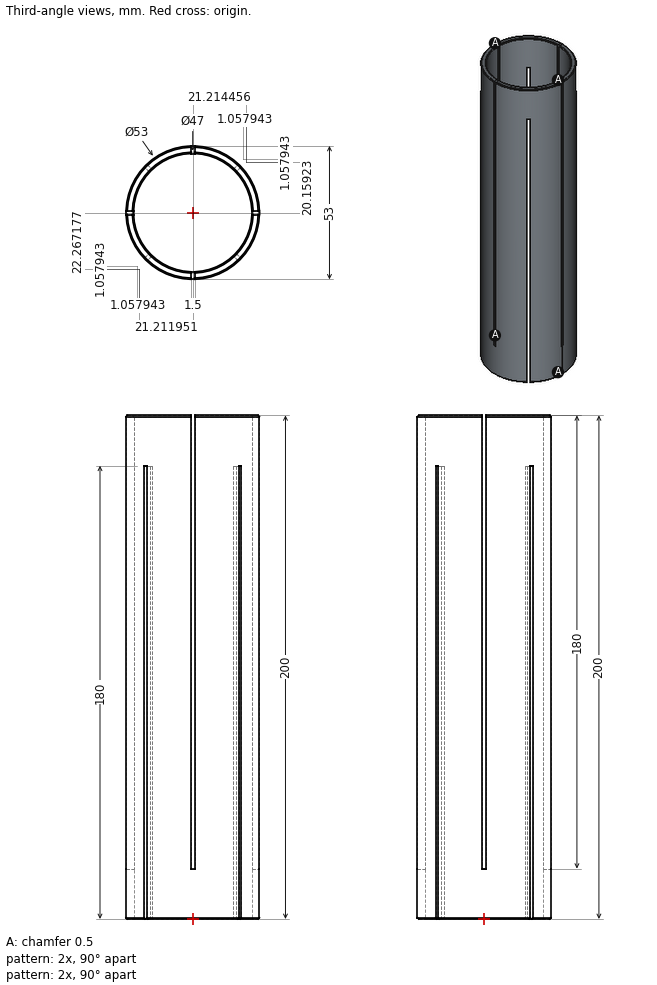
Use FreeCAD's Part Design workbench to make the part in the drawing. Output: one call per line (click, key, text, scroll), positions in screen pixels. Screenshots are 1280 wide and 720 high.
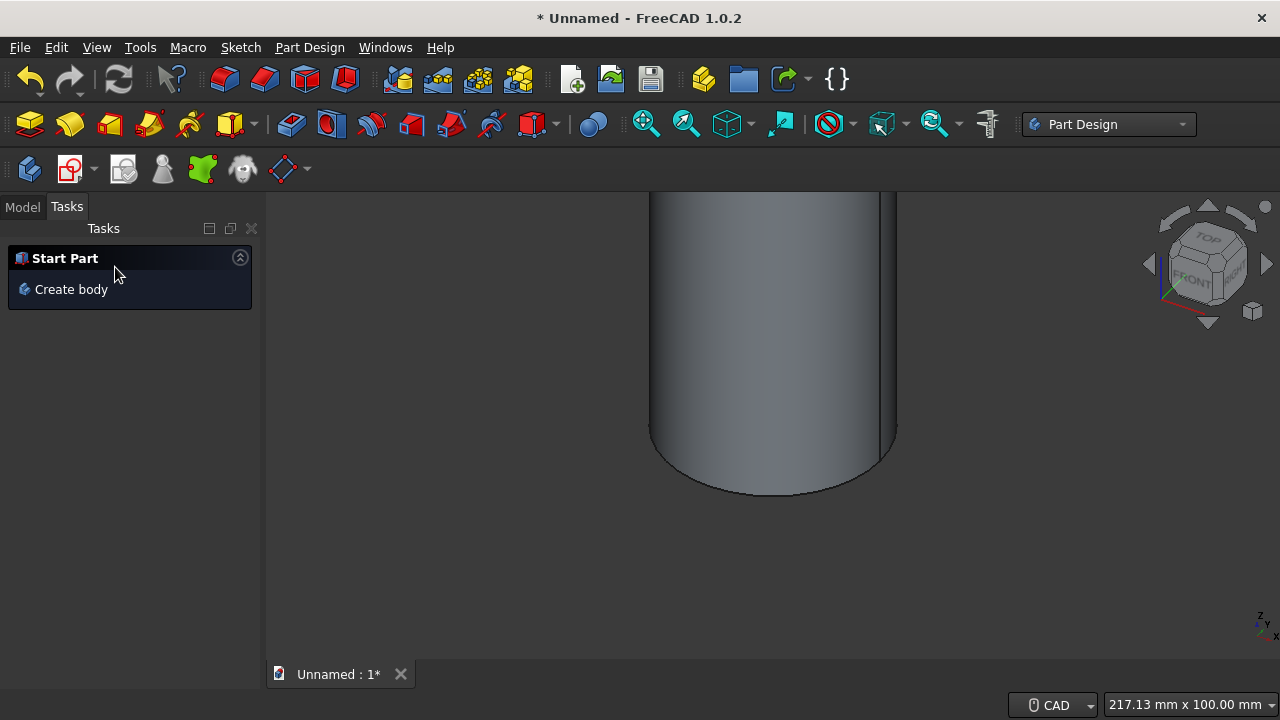
key(v)
key(f)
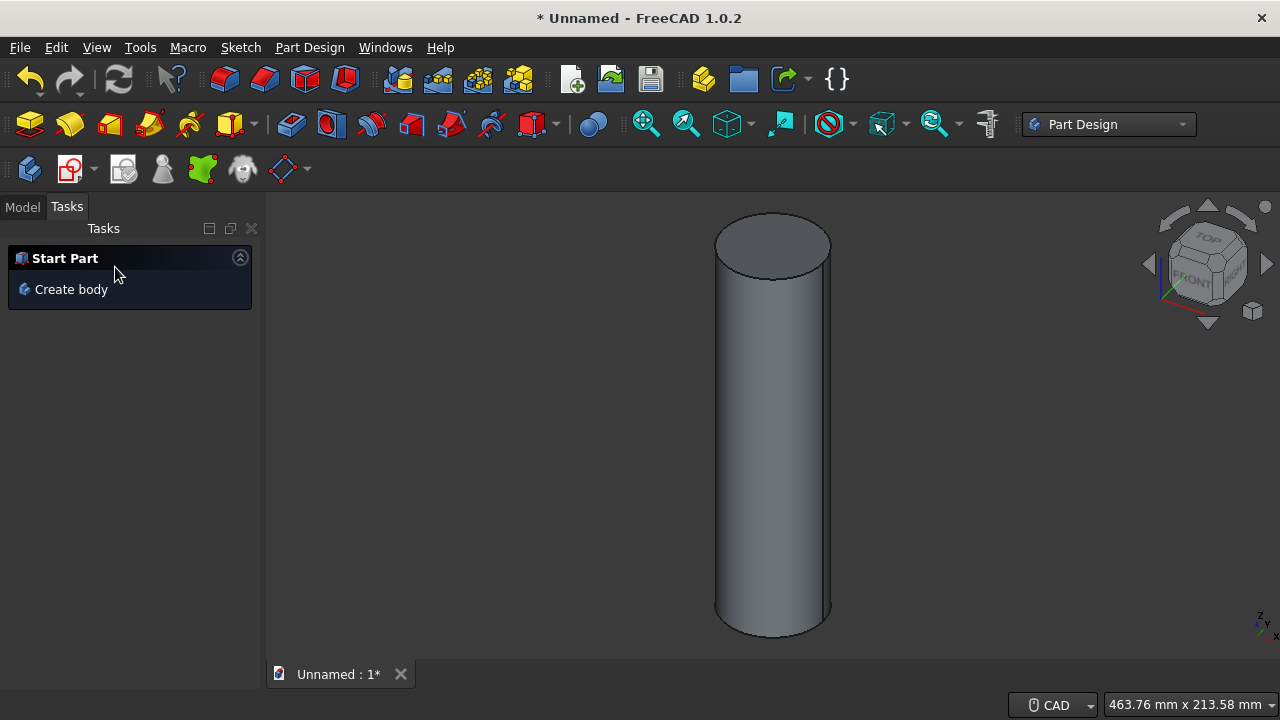
key(5)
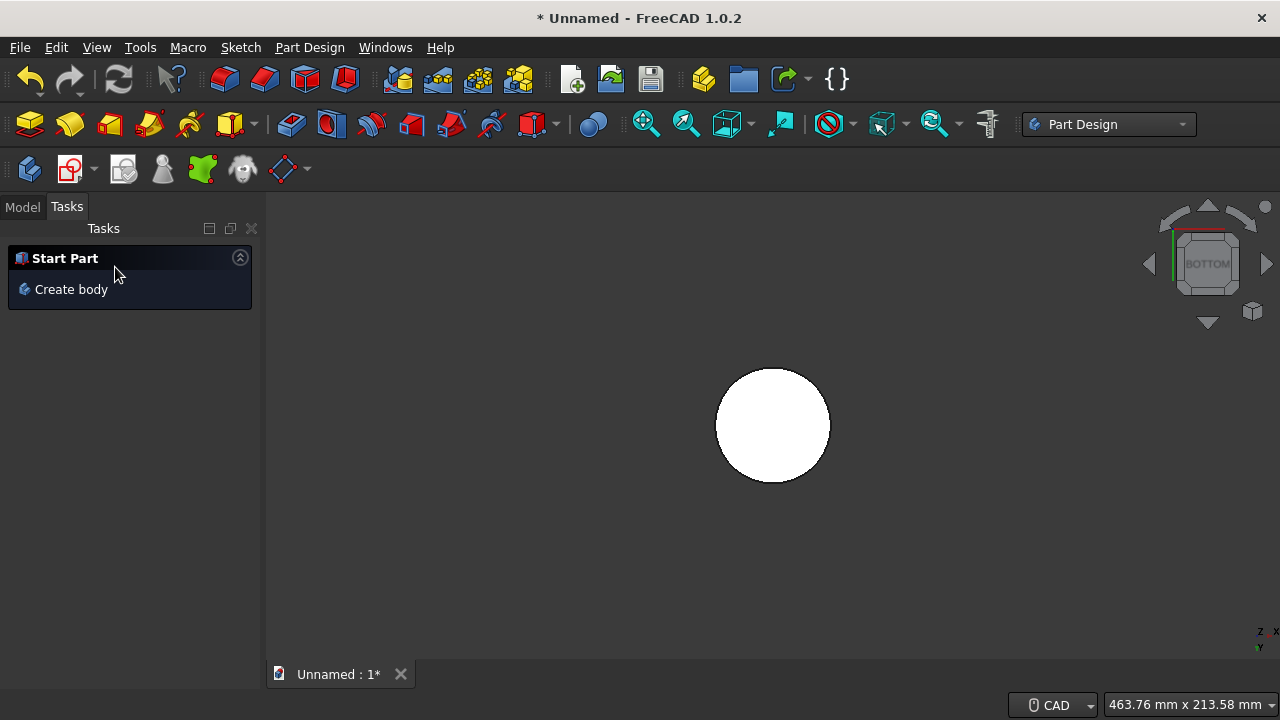
click(648, 124)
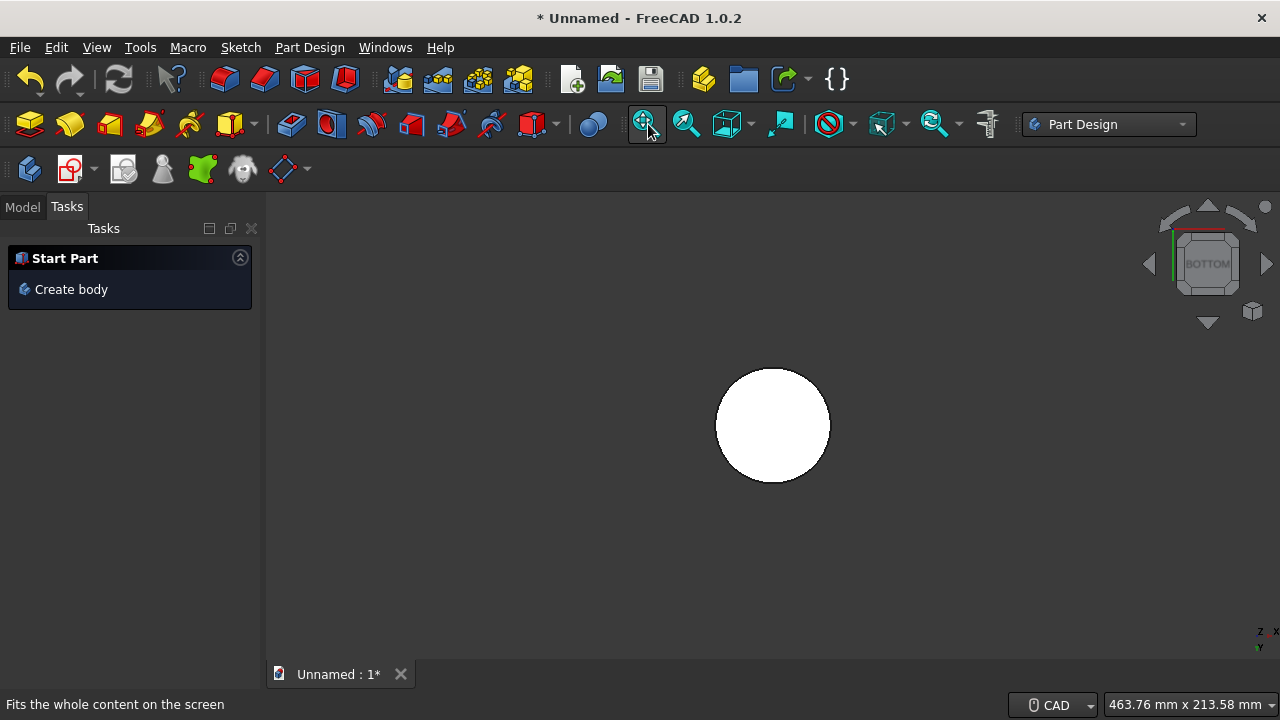
click(773, 424)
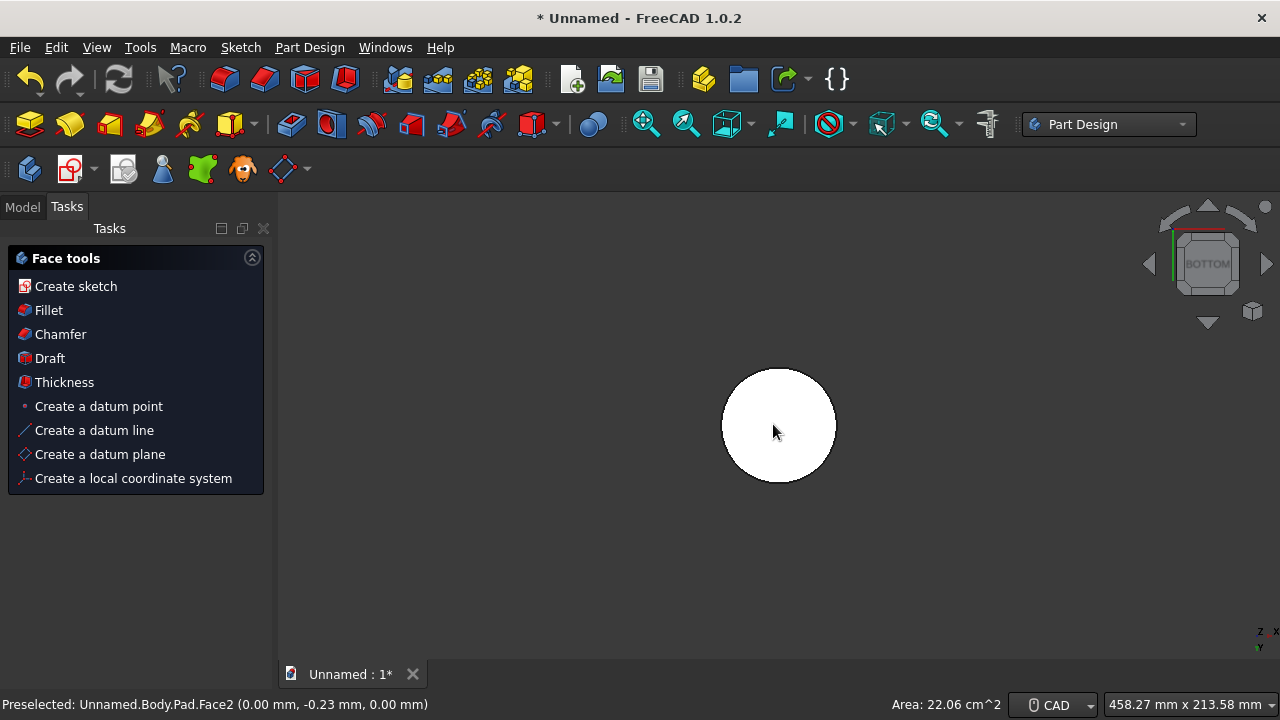
click(70, 170)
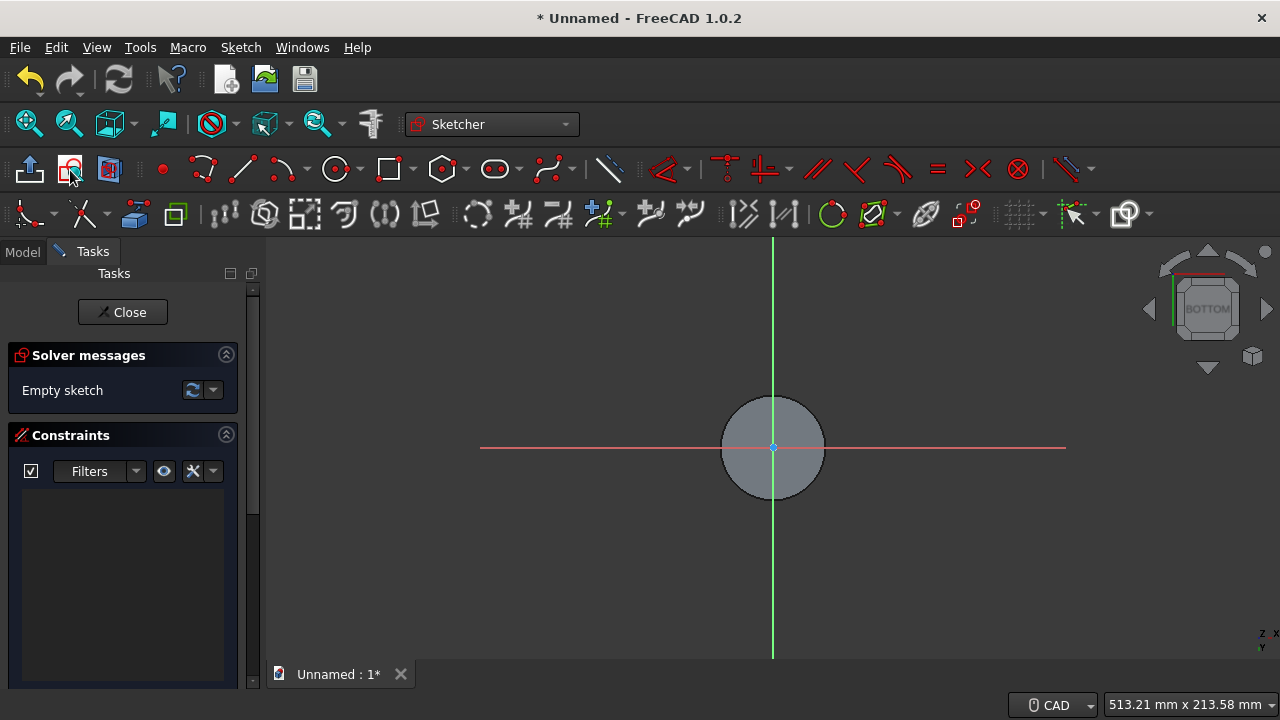
scroll(813, 448, up, 5)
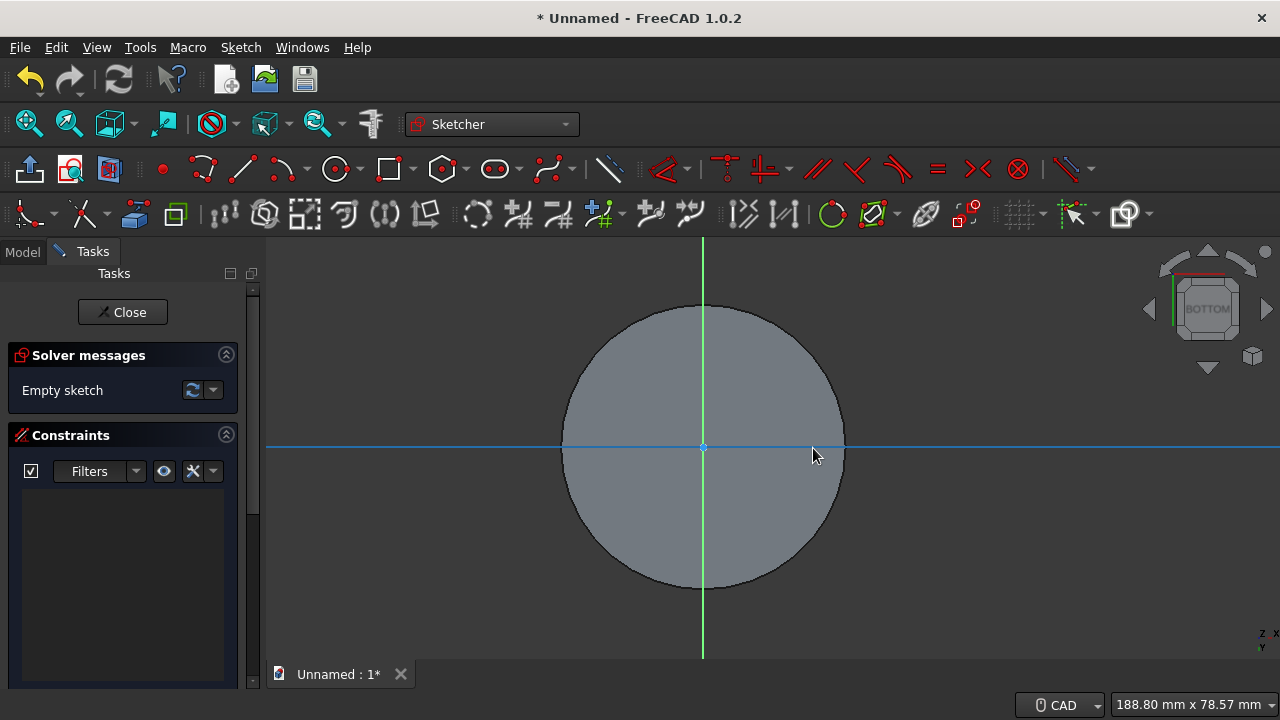
click(336, 170)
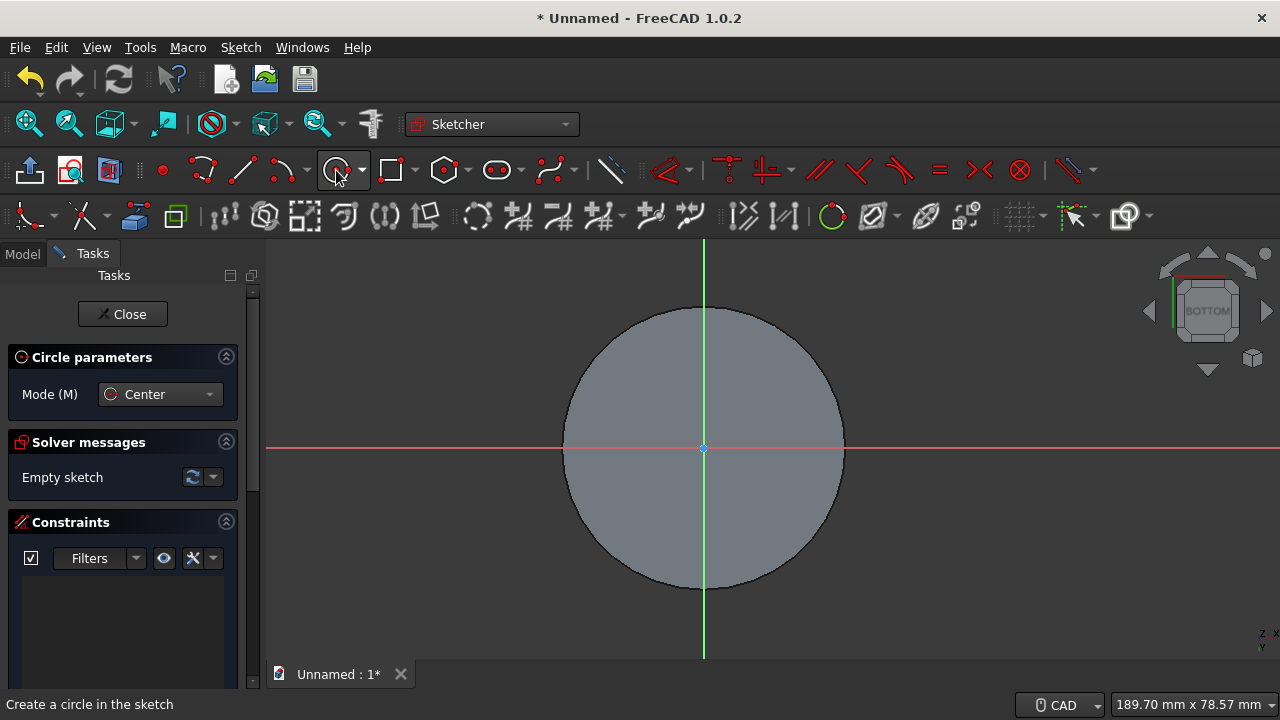
click(704, 448)
move(792, 359)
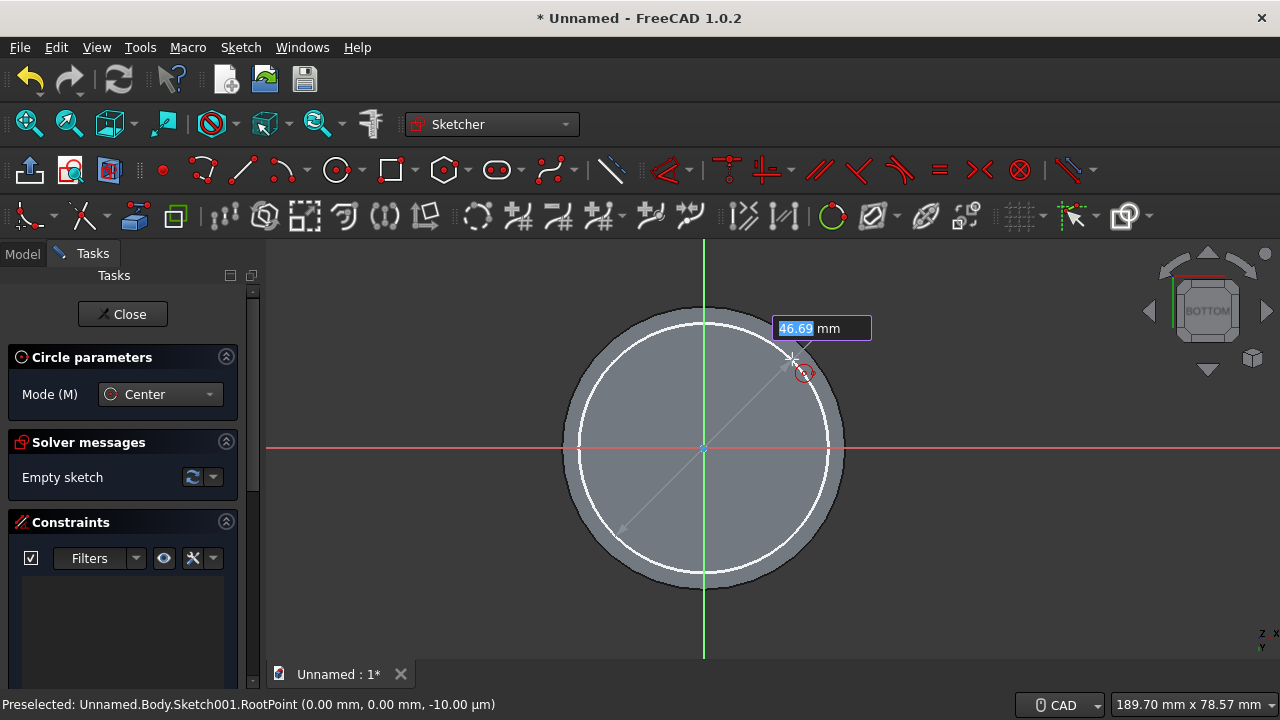
text(47)
key(Return)
key(Escape)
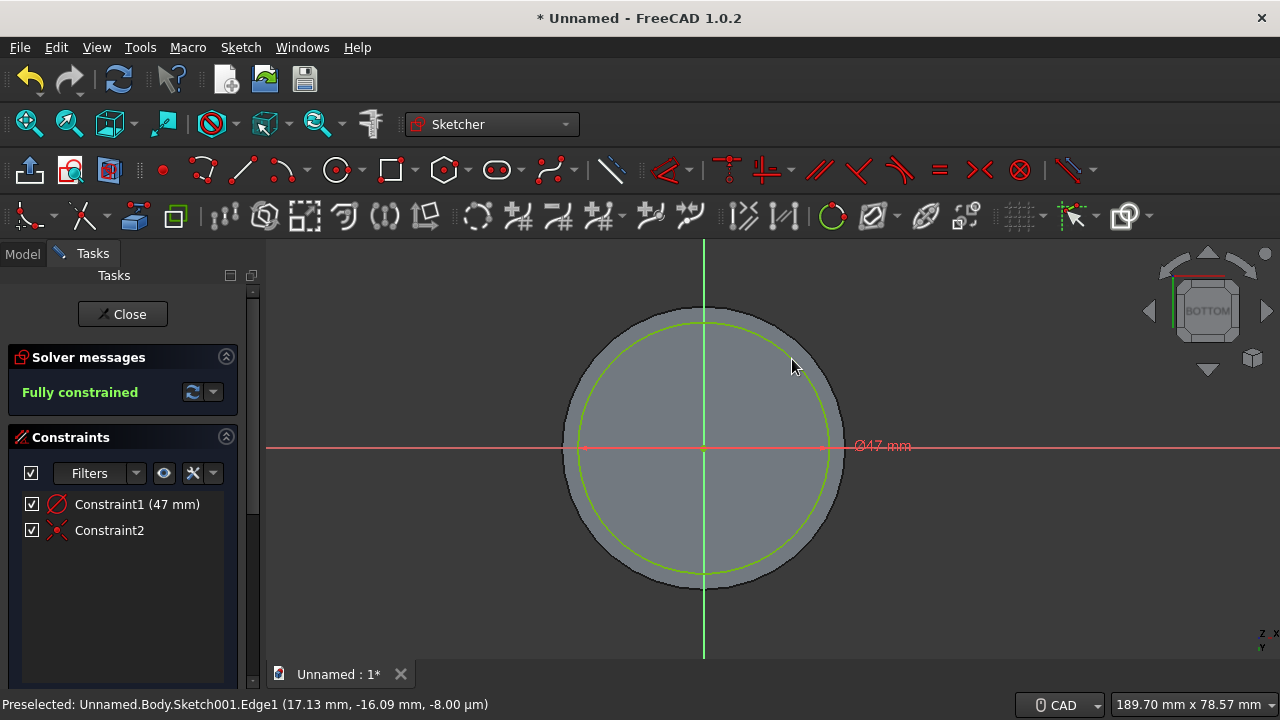
click(123, 314)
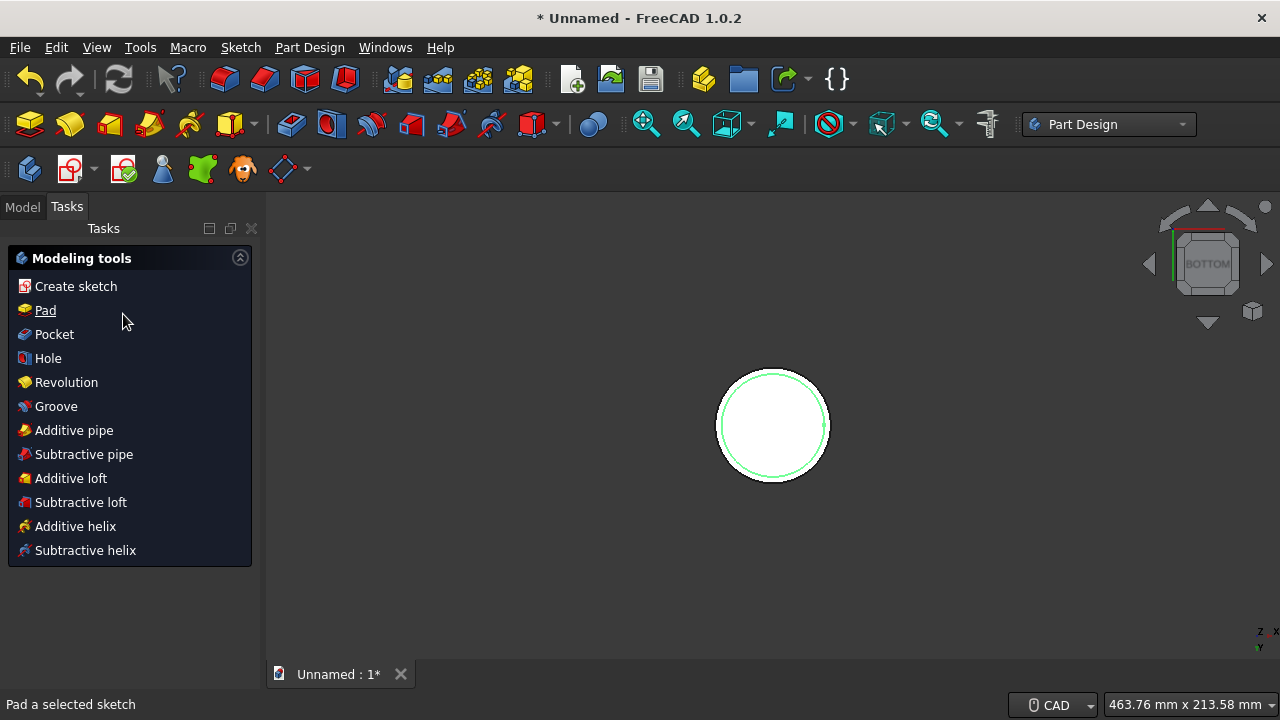
click(292, 124)